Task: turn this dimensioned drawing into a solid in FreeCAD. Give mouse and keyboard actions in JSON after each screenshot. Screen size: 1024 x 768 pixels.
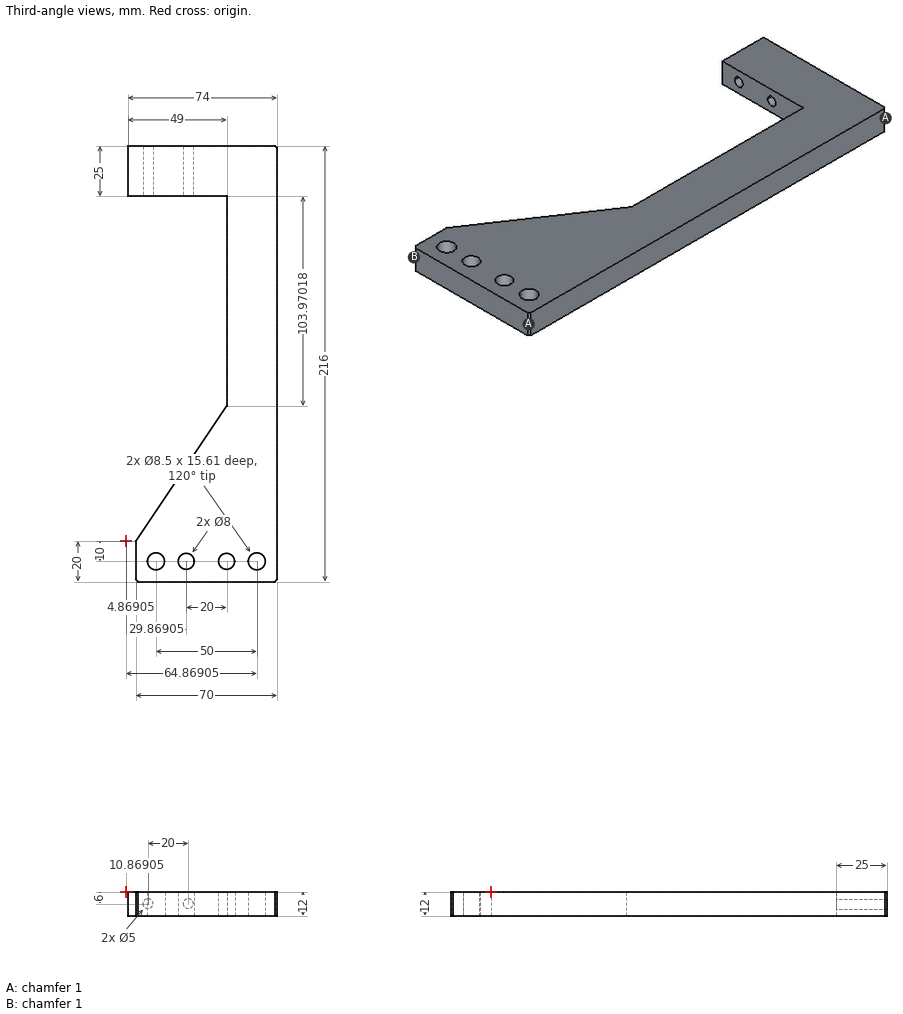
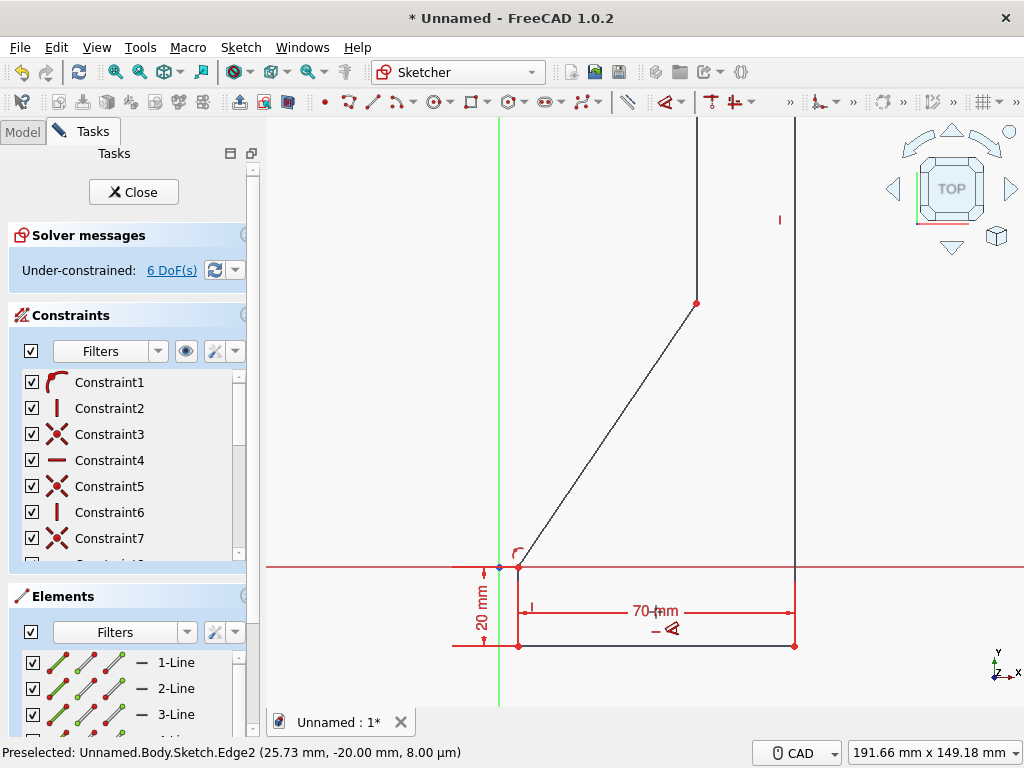
{"action": "scroll", "coordinate": [519, 569], "scroll_direction": "down", "scroll_amount": 4}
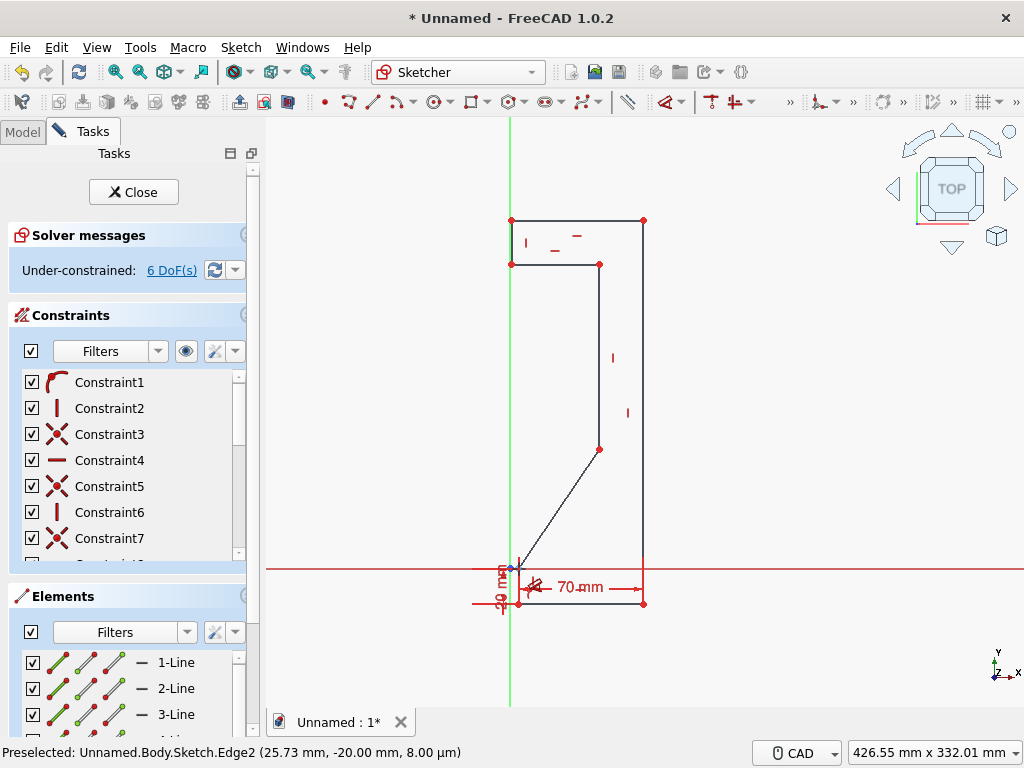
{"action": "left_click", "coordinate": [604, 221]}
{"action": "left_click", "coordinate": [577, 187]}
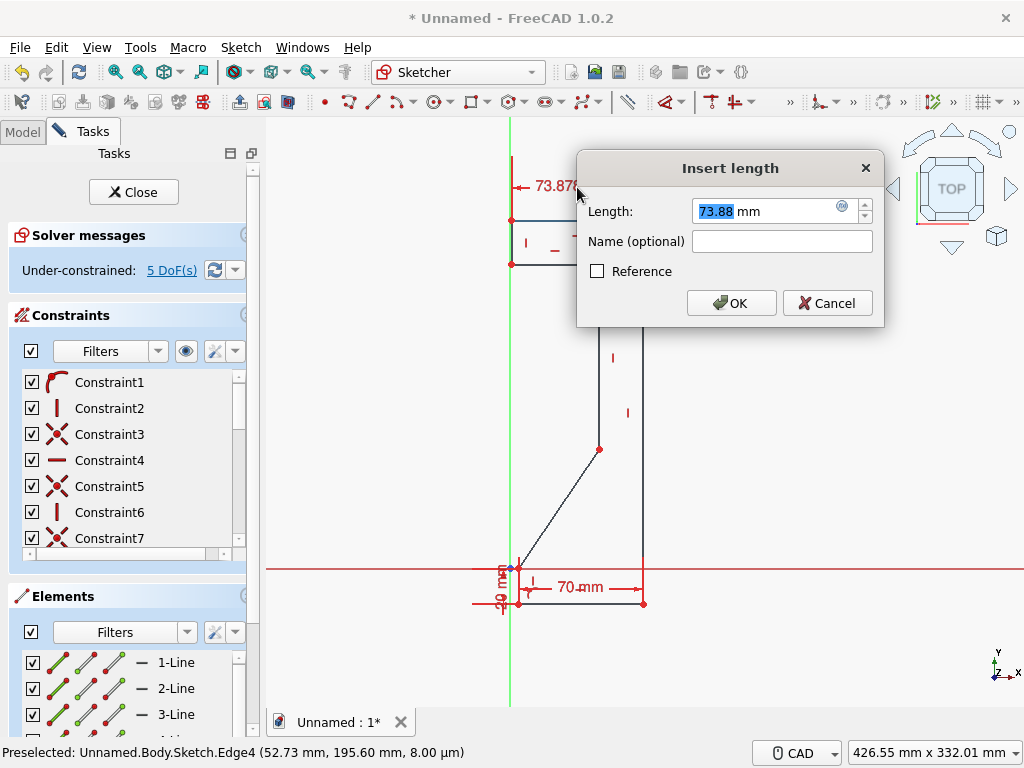
{"action": "type", "text": "74"}
{"action": "key", "text": "Return"}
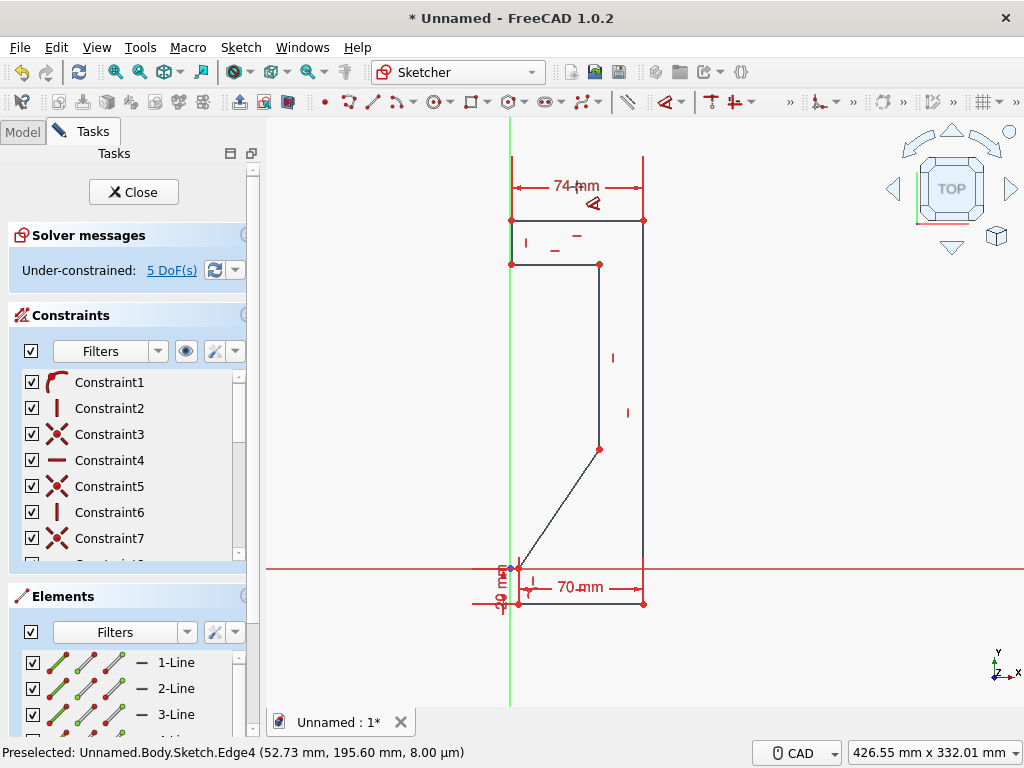
{"action": "left_click", "coordinate": [512, 234]}
{"action": "left_click", "coordinate": [478, 243]}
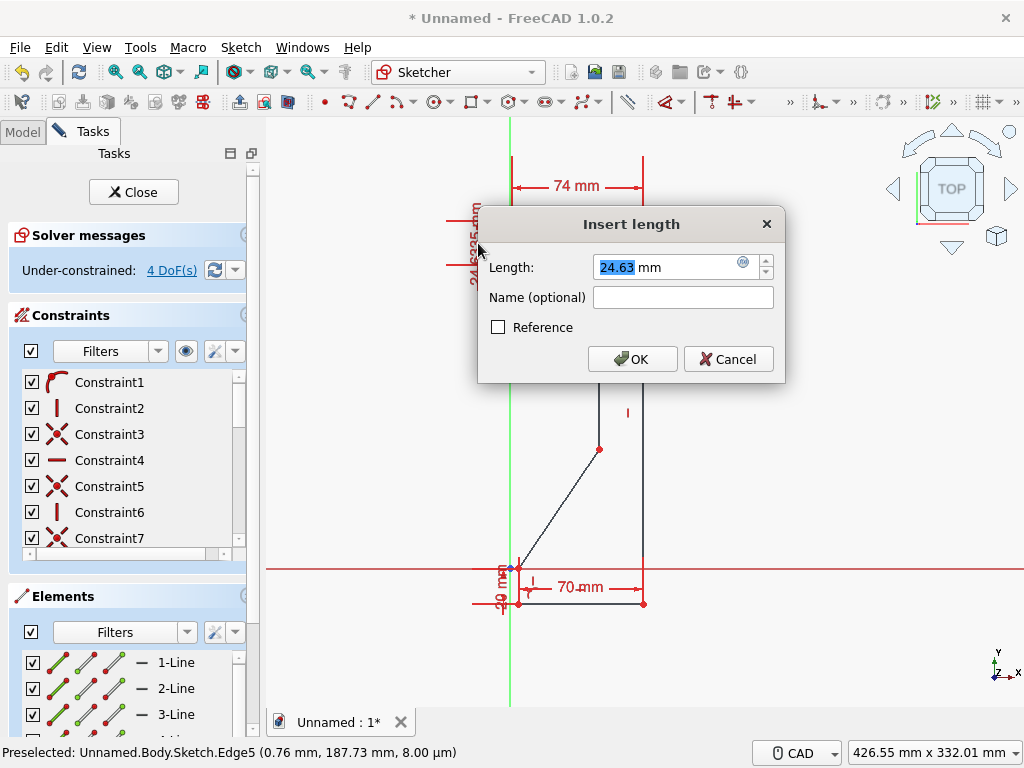
{"action": "type", "text": "25"}
{"action": "key", "text": "Return"}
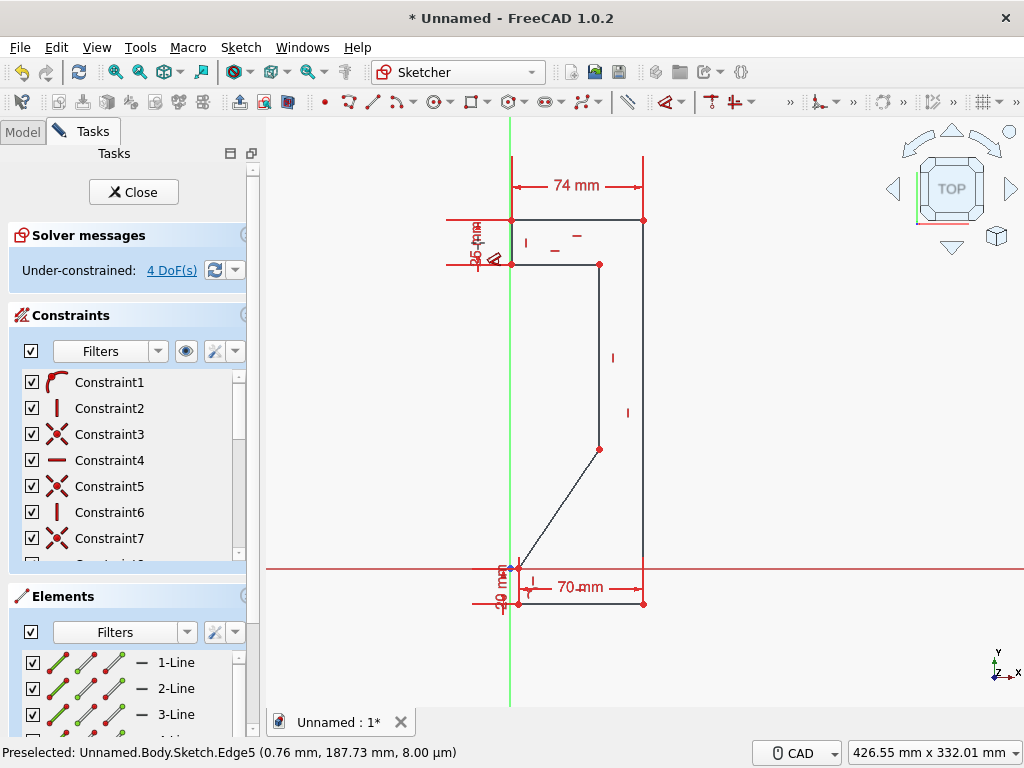
{"action": "left_click", "coordinate": [538, 265]}
{"action": "left_click", "coordinate": [555, 299]}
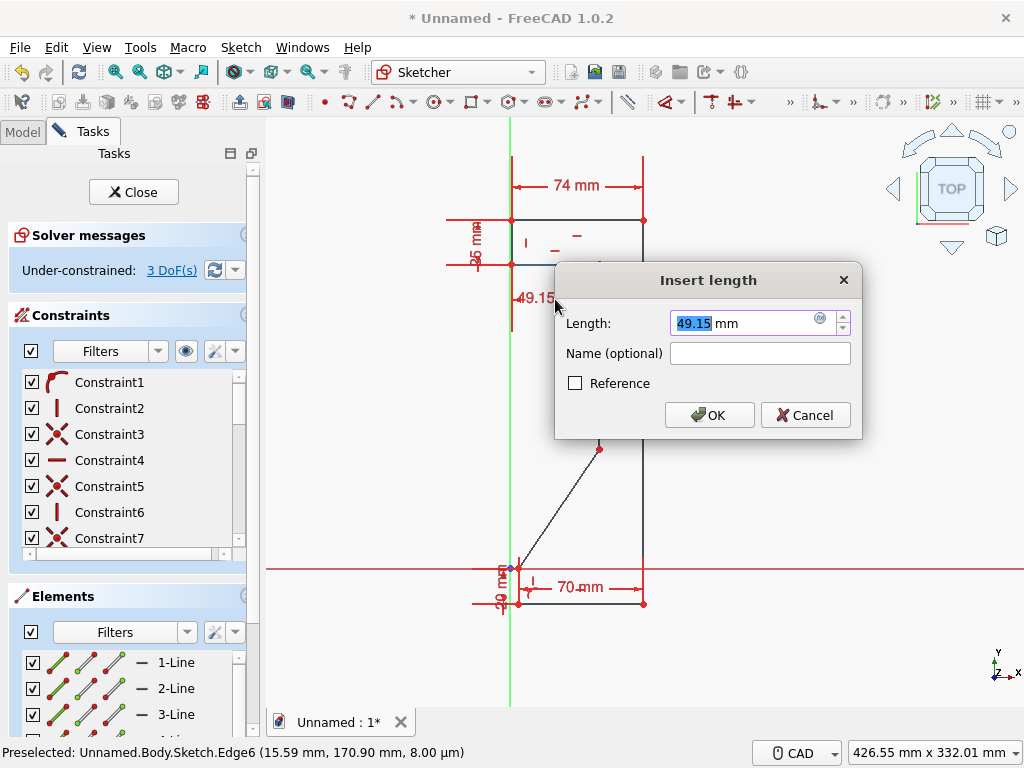
{"action": "type", "text": "49"}
{"action": "key", "text": "Return"}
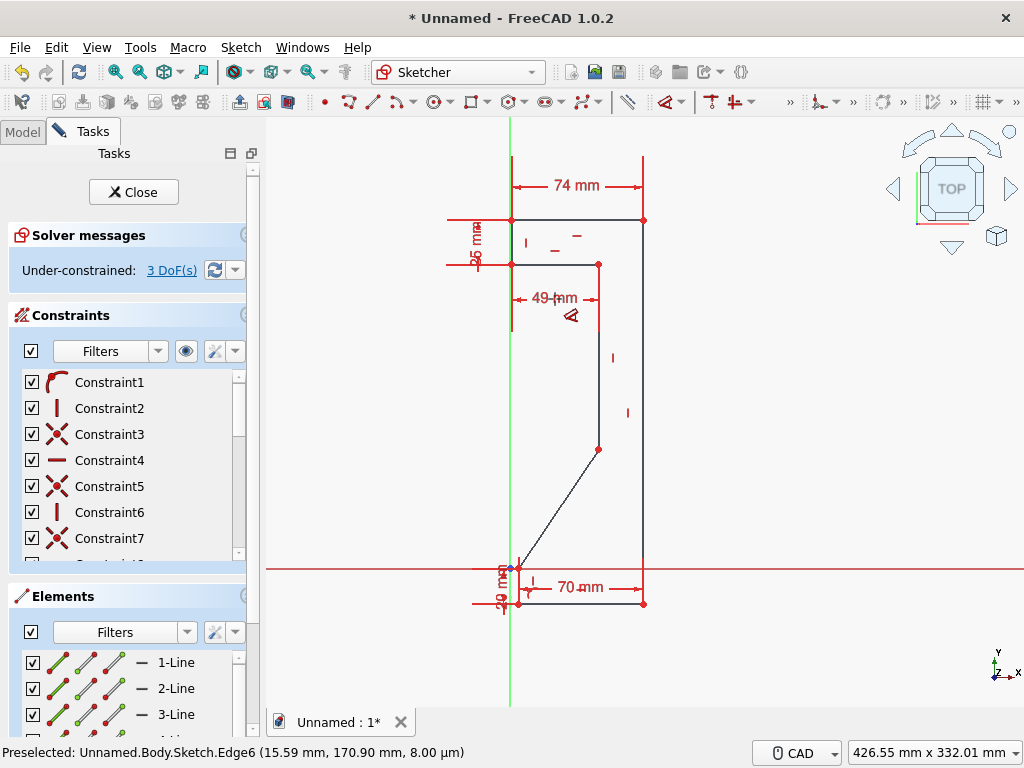
{"action": "left_click", "coordinate": [643, 489]}
{"action": "left_click", "coordinate": [677, 412]}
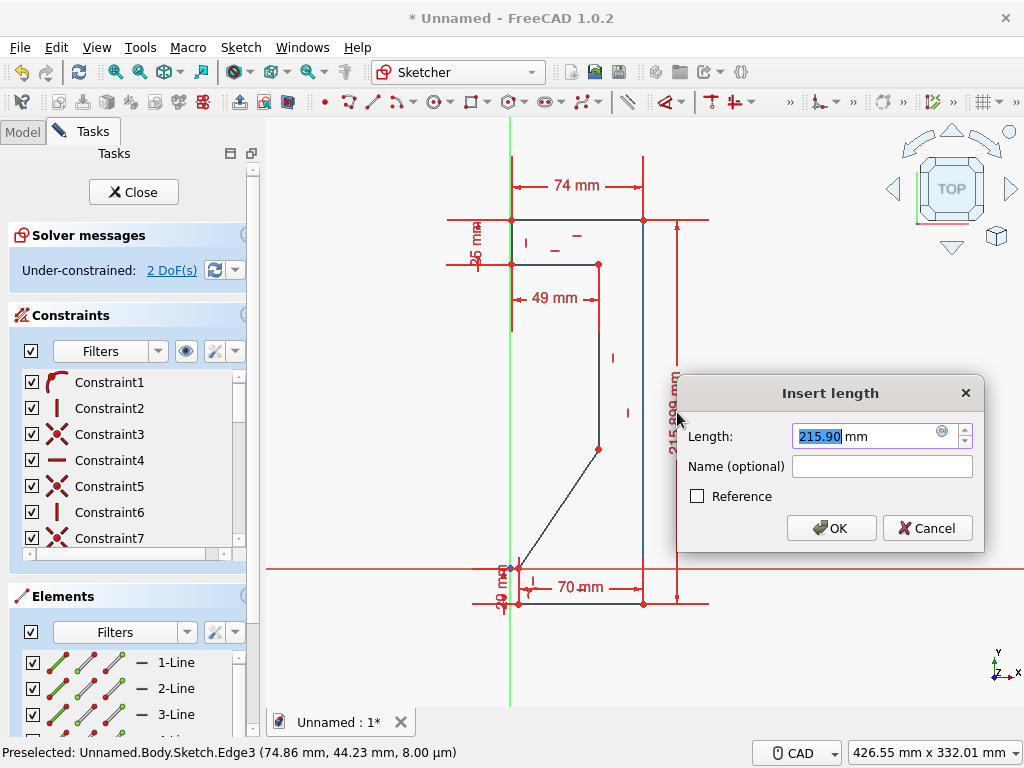
{"action": "type", "text": "216"}
{"action": "key", "text": "Return"}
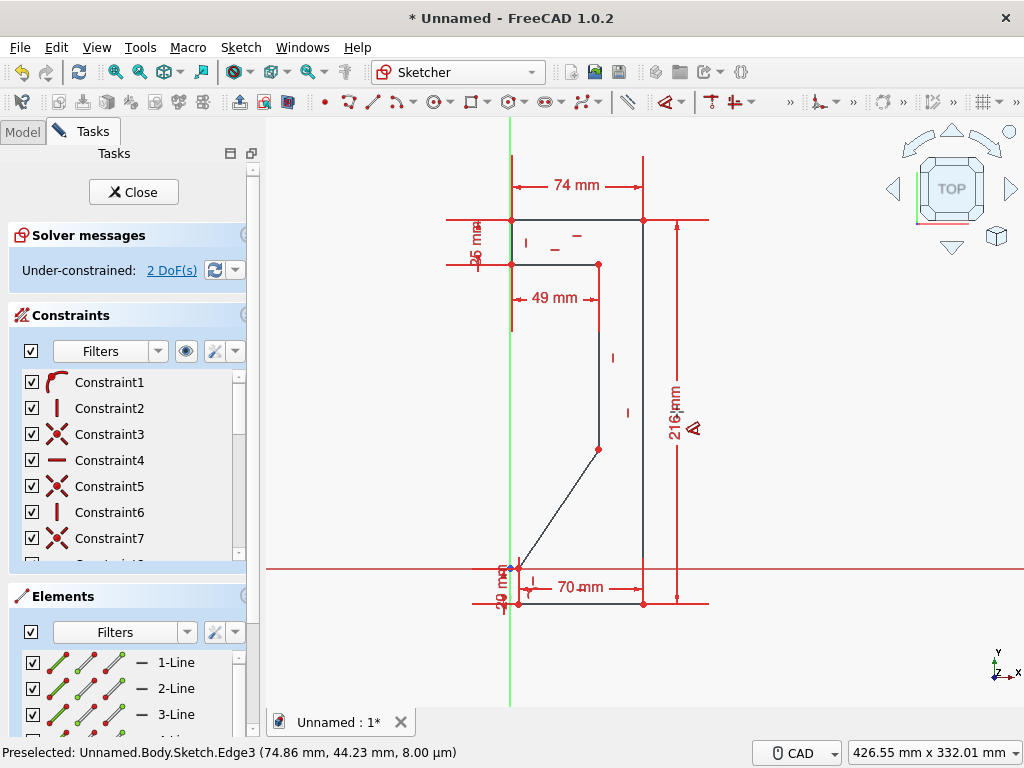
{"action": "scroll", "coordinate": [519, 569], "scroll_direction": "up", "scroll_amount": 8}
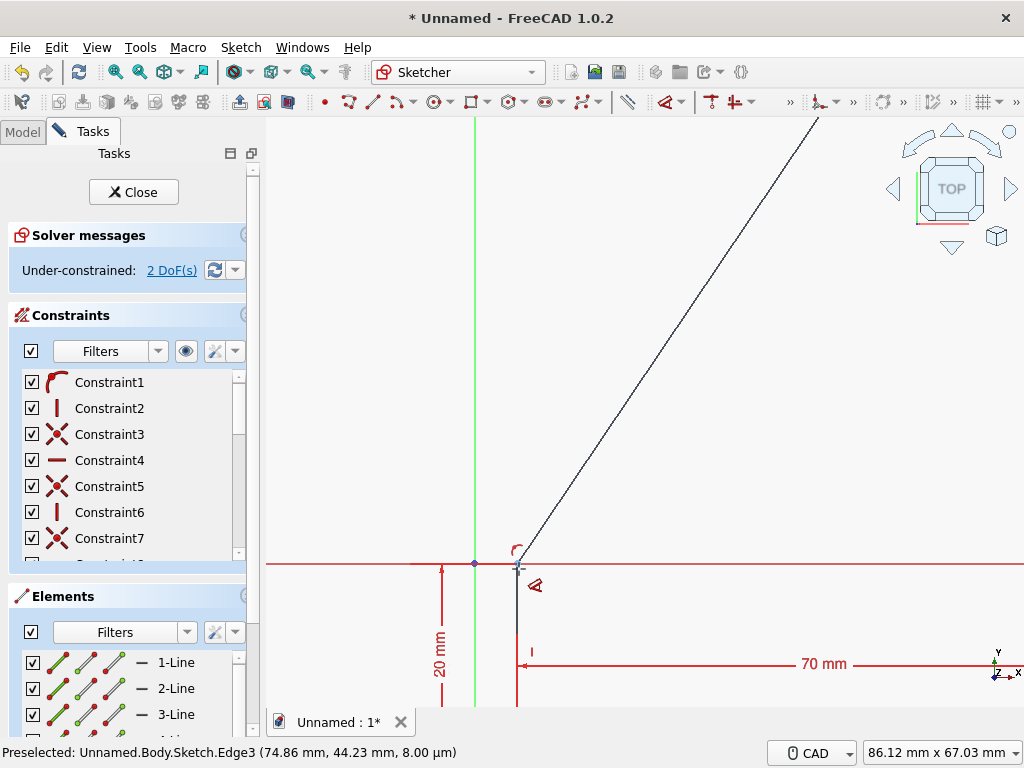
{"action": "left_click", "coordinate": [517, 564]}
{"action": "left_click", "coordinate": [496, 598]}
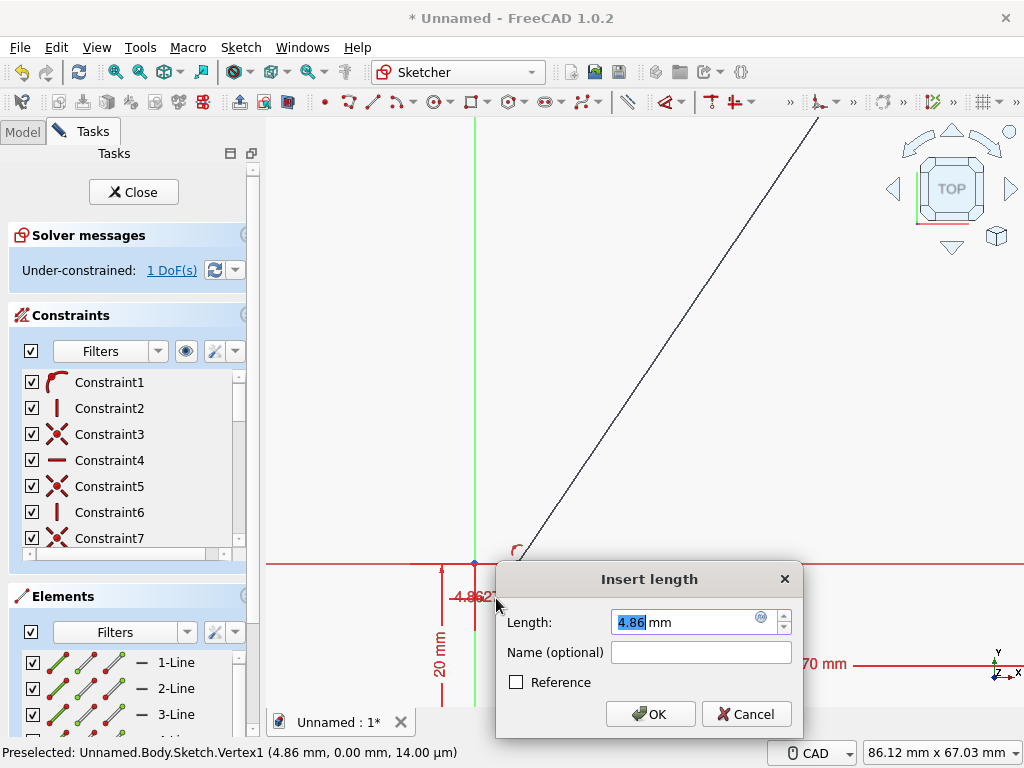
{"action": "type", "text": "4.86905"}
{"action": "key", "text": "Return"}